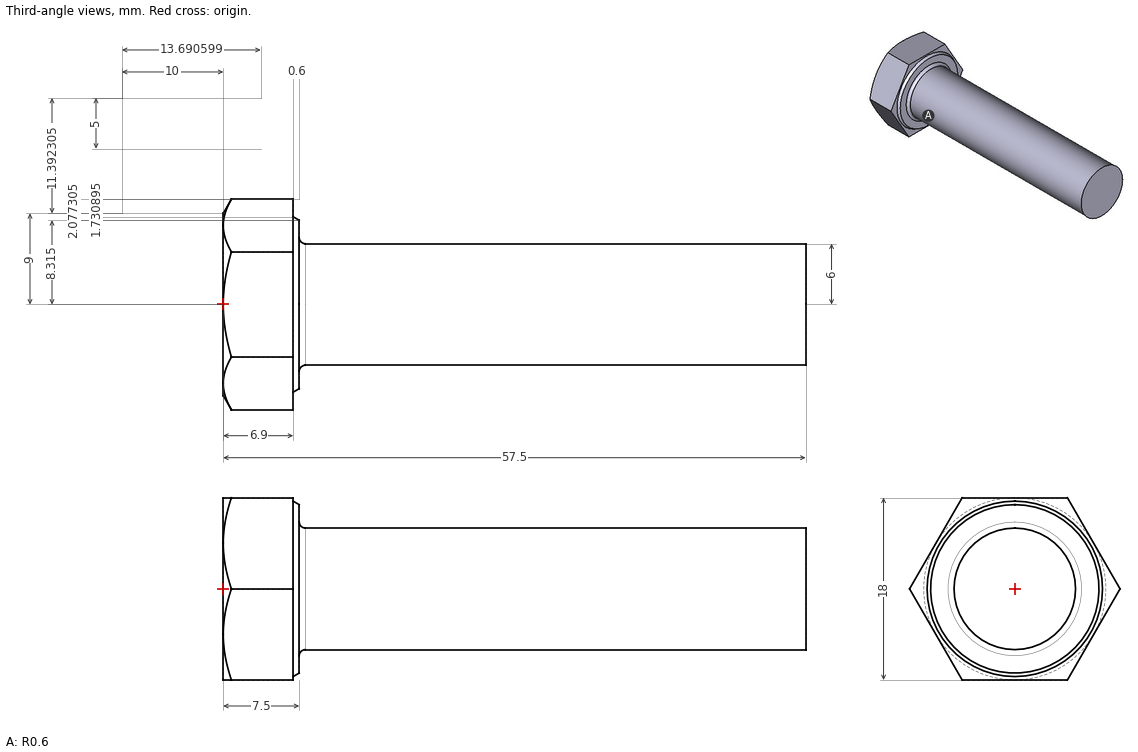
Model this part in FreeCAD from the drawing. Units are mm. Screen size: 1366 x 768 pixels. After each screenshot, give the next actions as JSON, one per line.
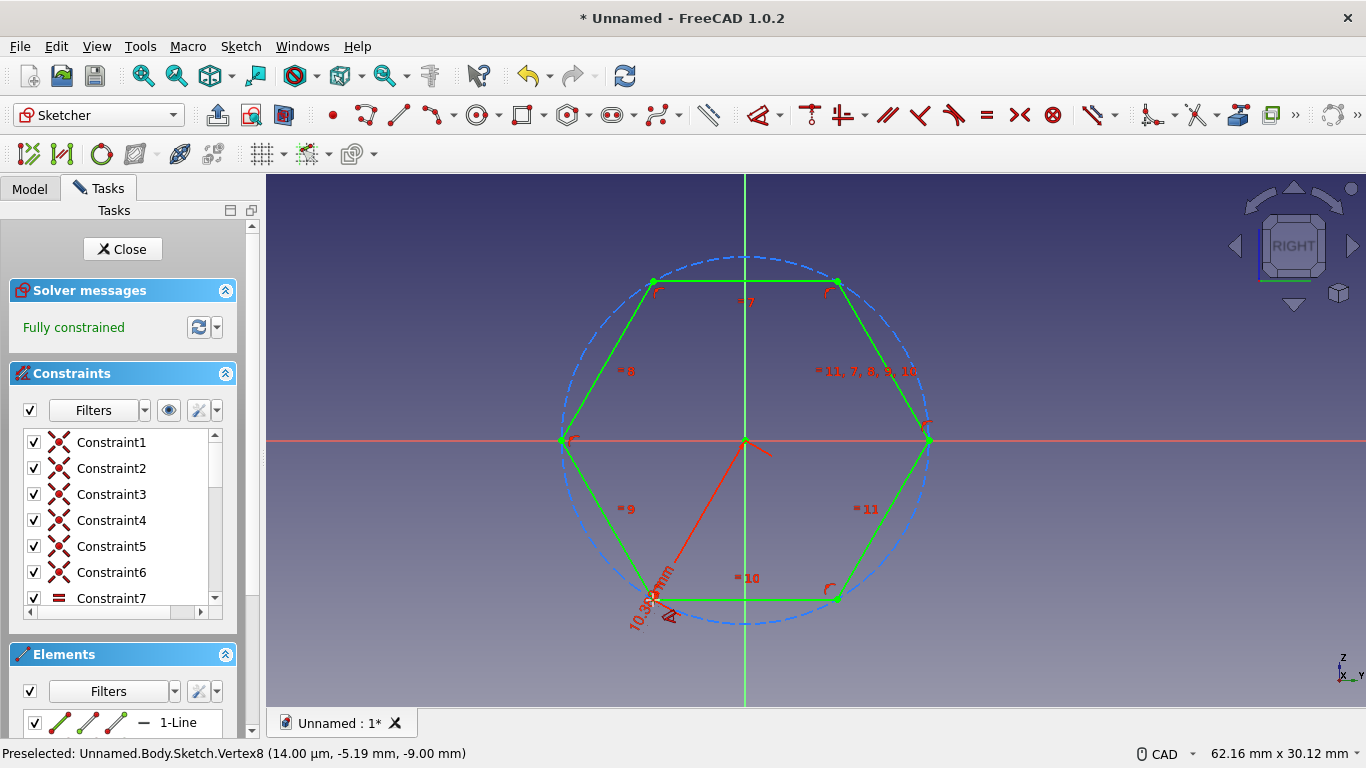
{"action": "left_click", "coordinate": [837, 281]}
{"action": "left_click", "coordinate": [871, 367]}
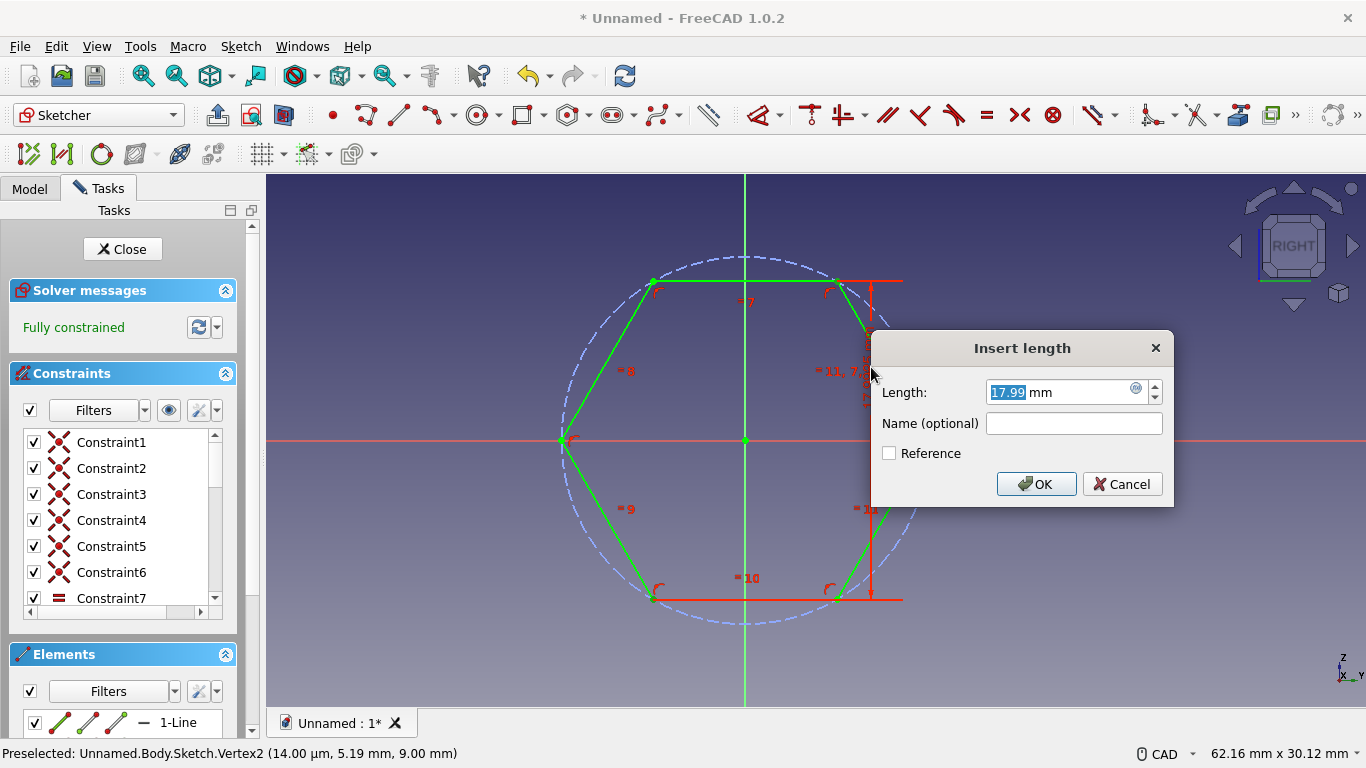
{"action": "type", "text": "18"}
{"action": "key", "text": "Return"}
{"action": "key", "text": "Escape"}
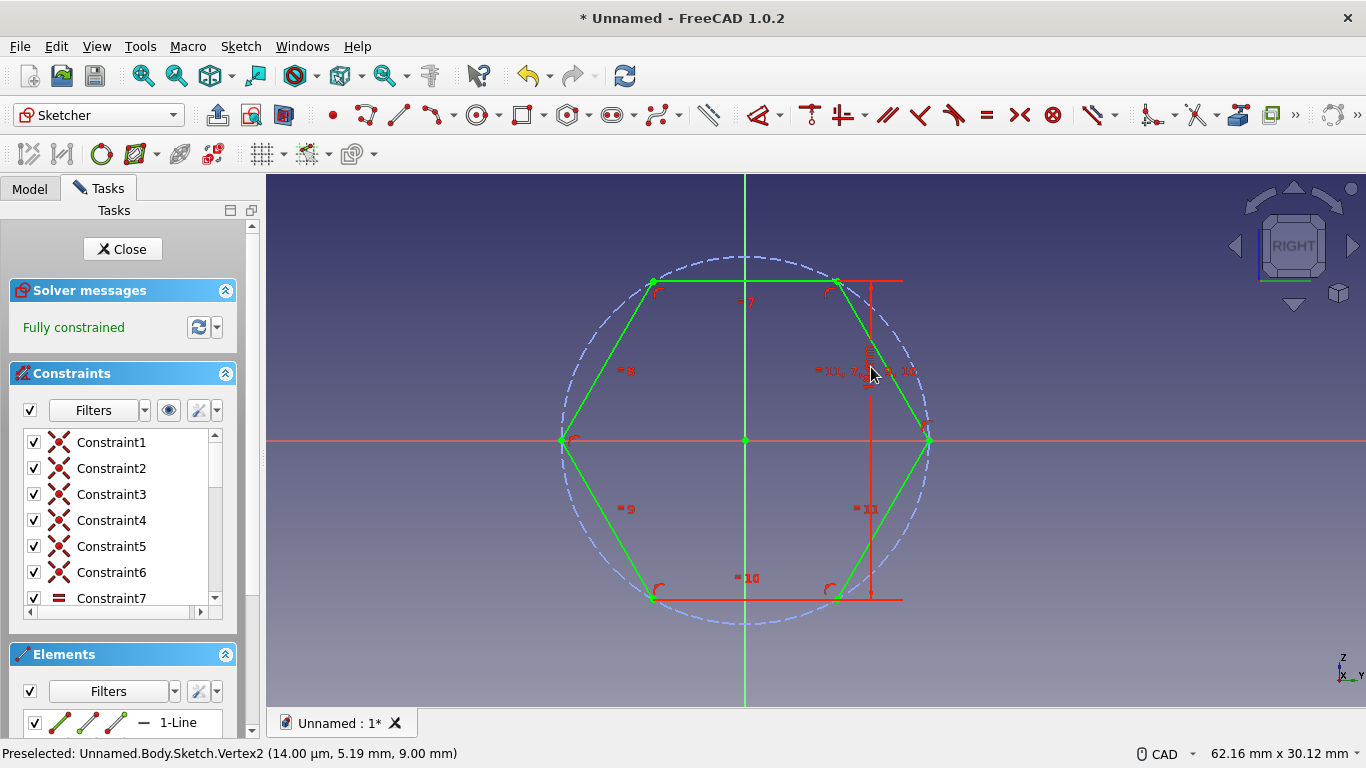
{"action": "left_click", "coordinate": [123, 249]}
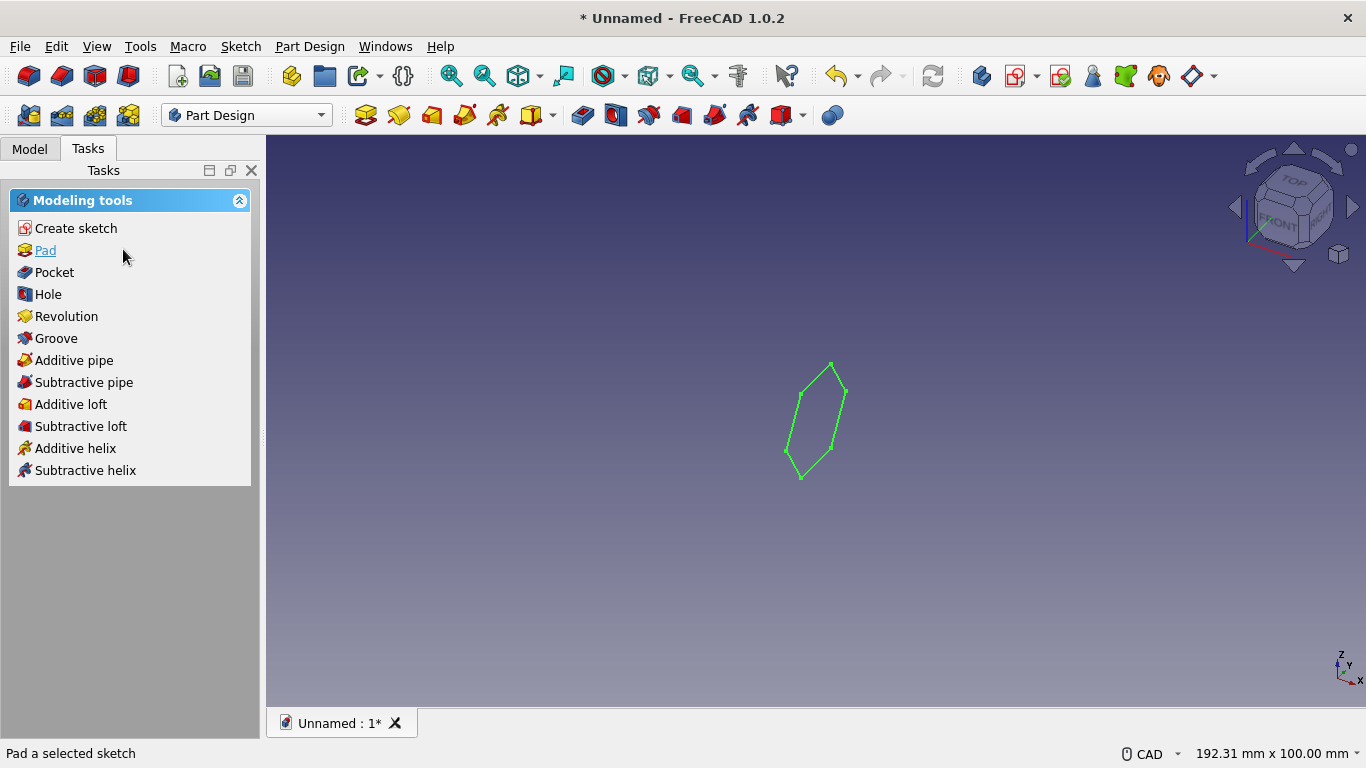
{"action": "left_click", "coordinate": [366, 116]}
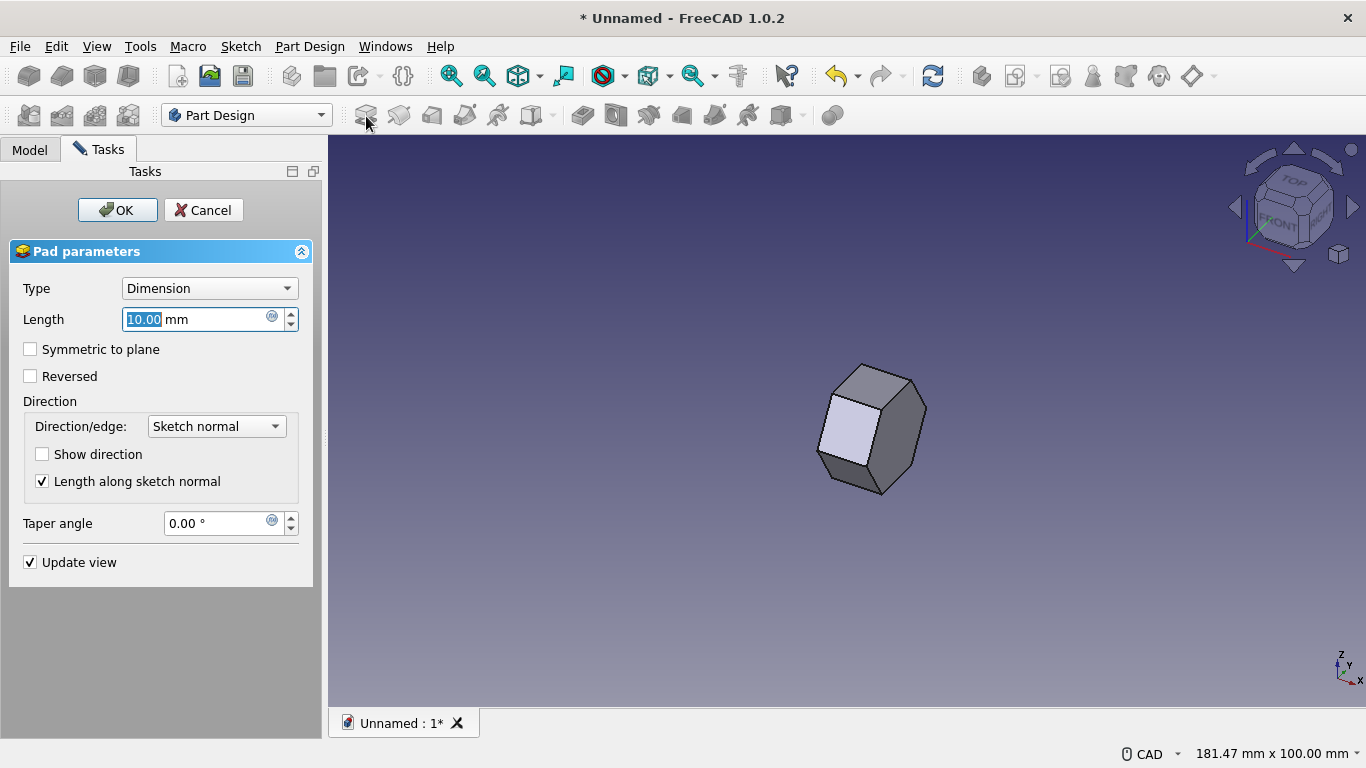
{"action": "type", "text": "7.5"}
{"action": "key", "text": "Tab"}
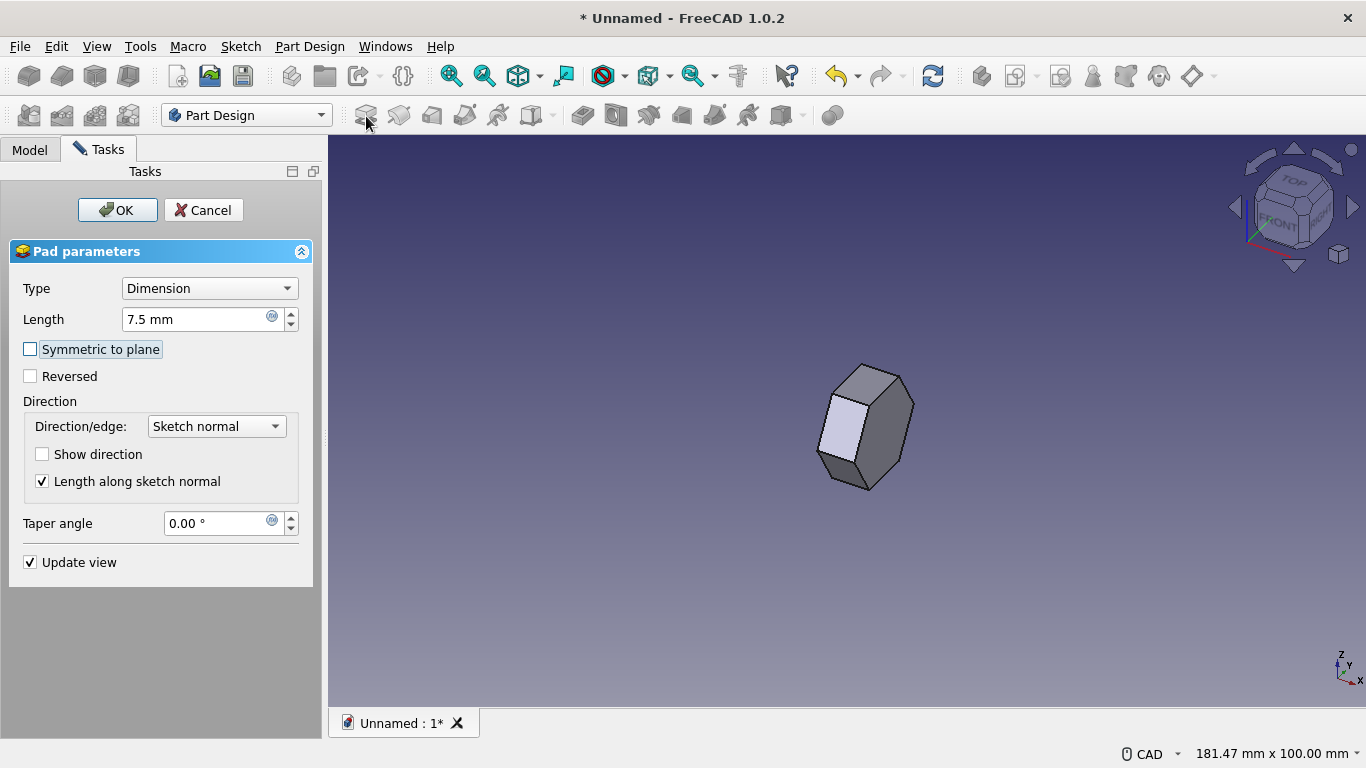
{"action": "left_click", "coordinate": [118, 210]}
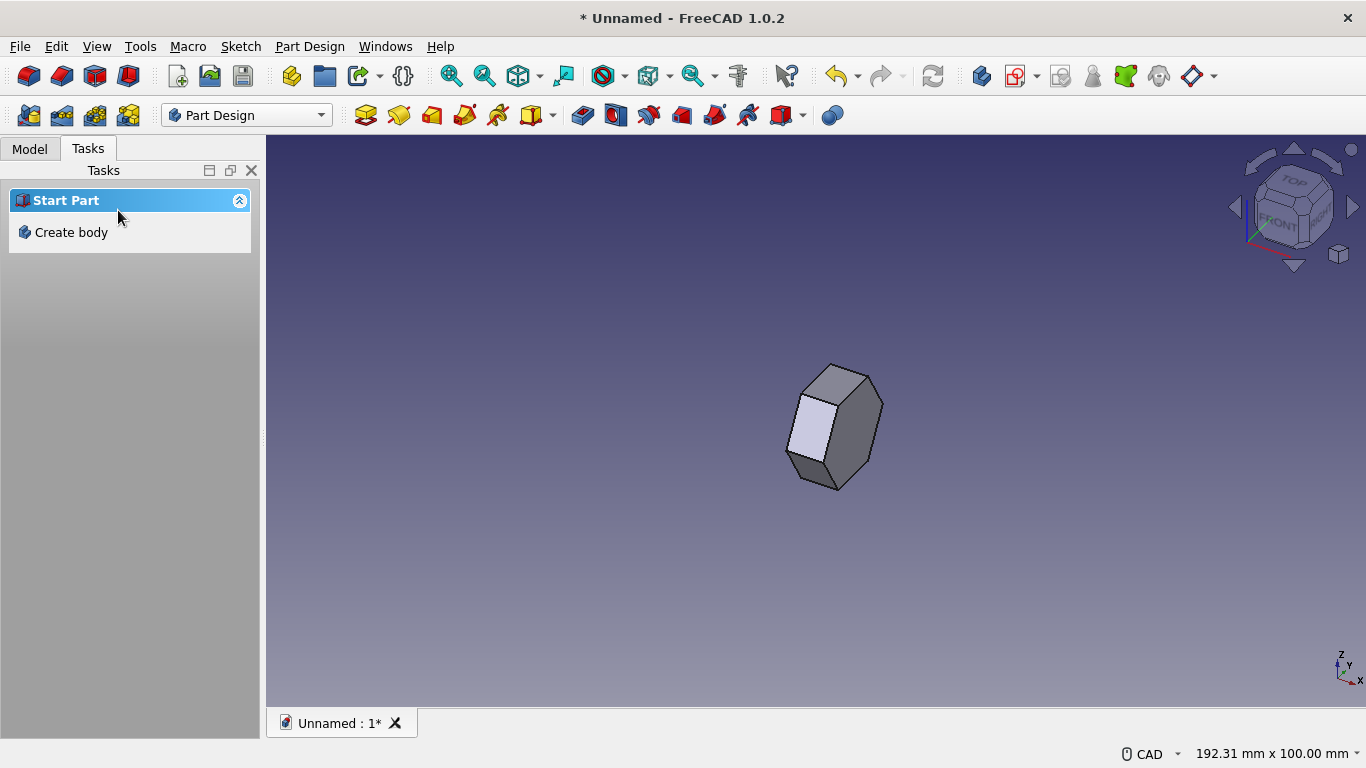
{"action": "left_click", "coordinate": [452, 76]}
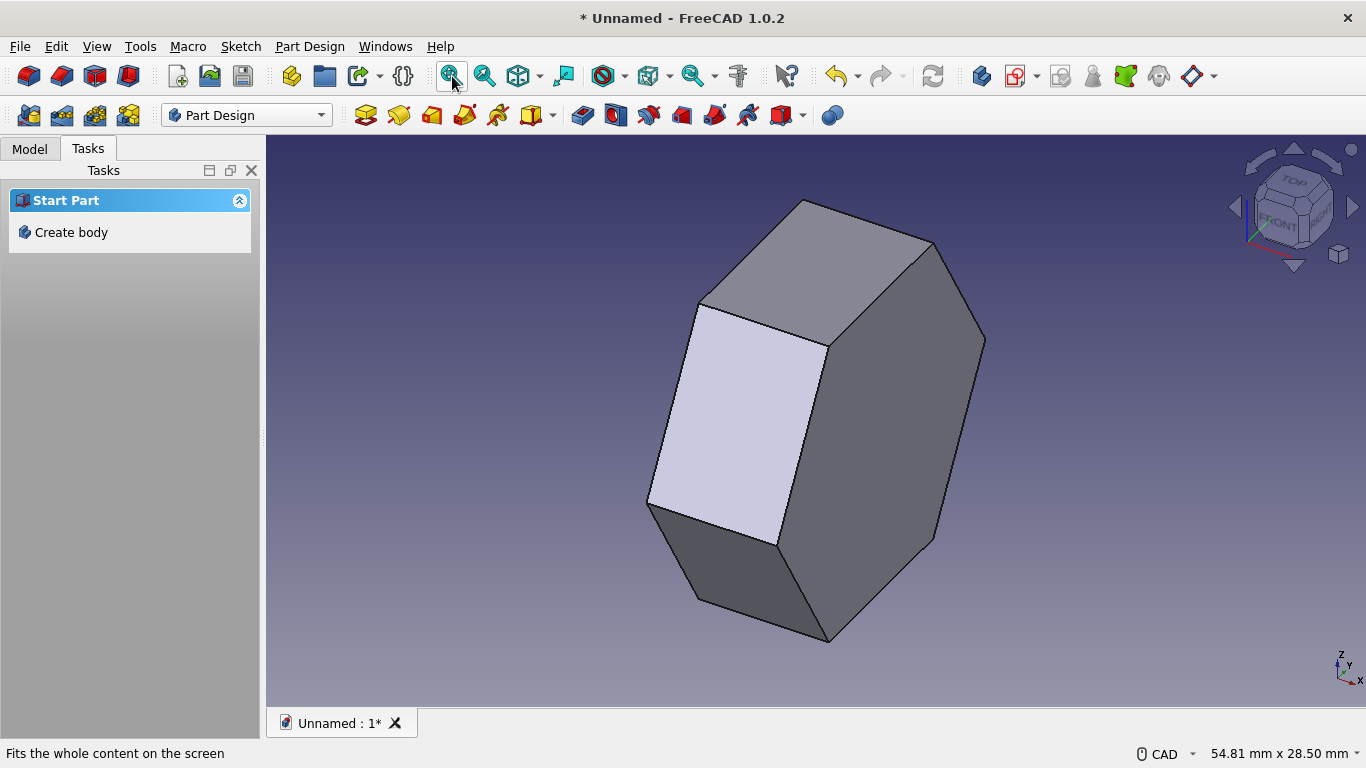
{"action": "left_click", "coordinate": [1014, 76]}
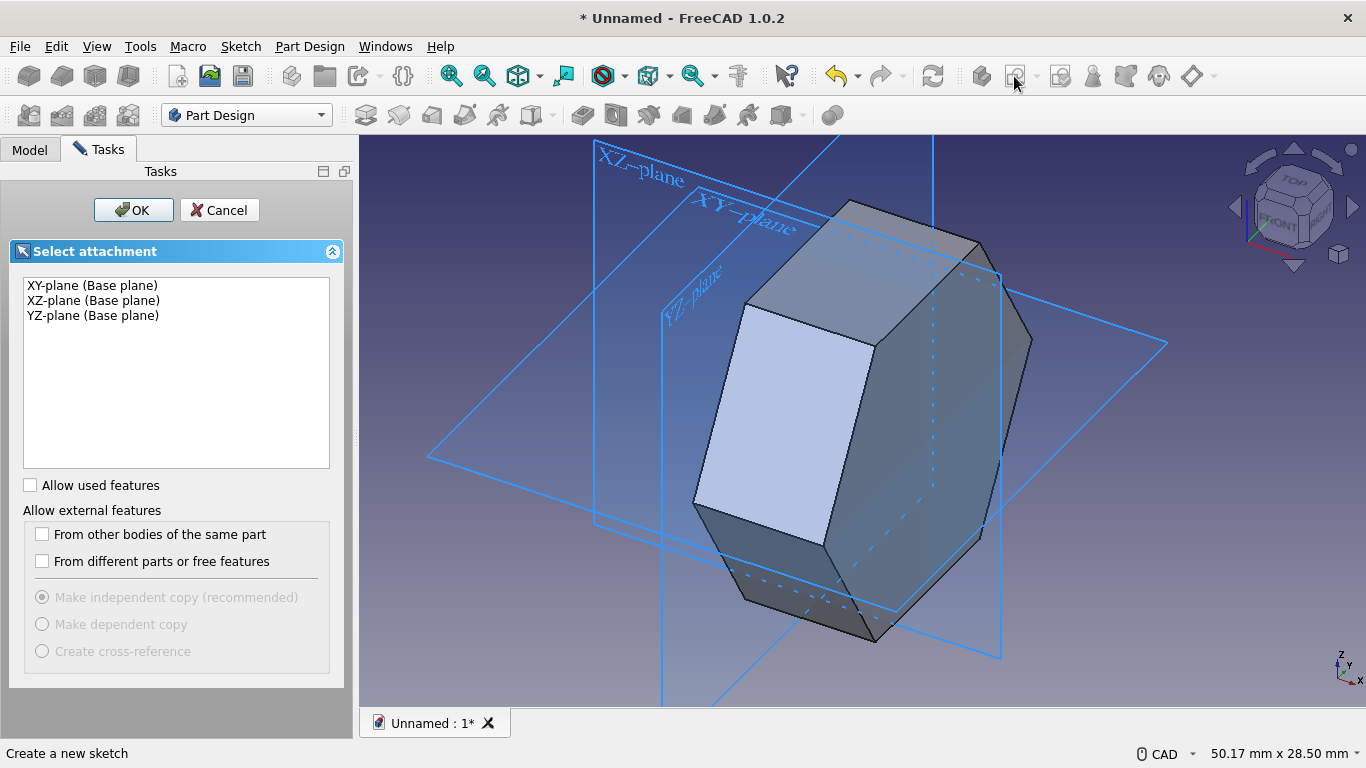
{"action": "left_click", "coordinate": [84, 286]}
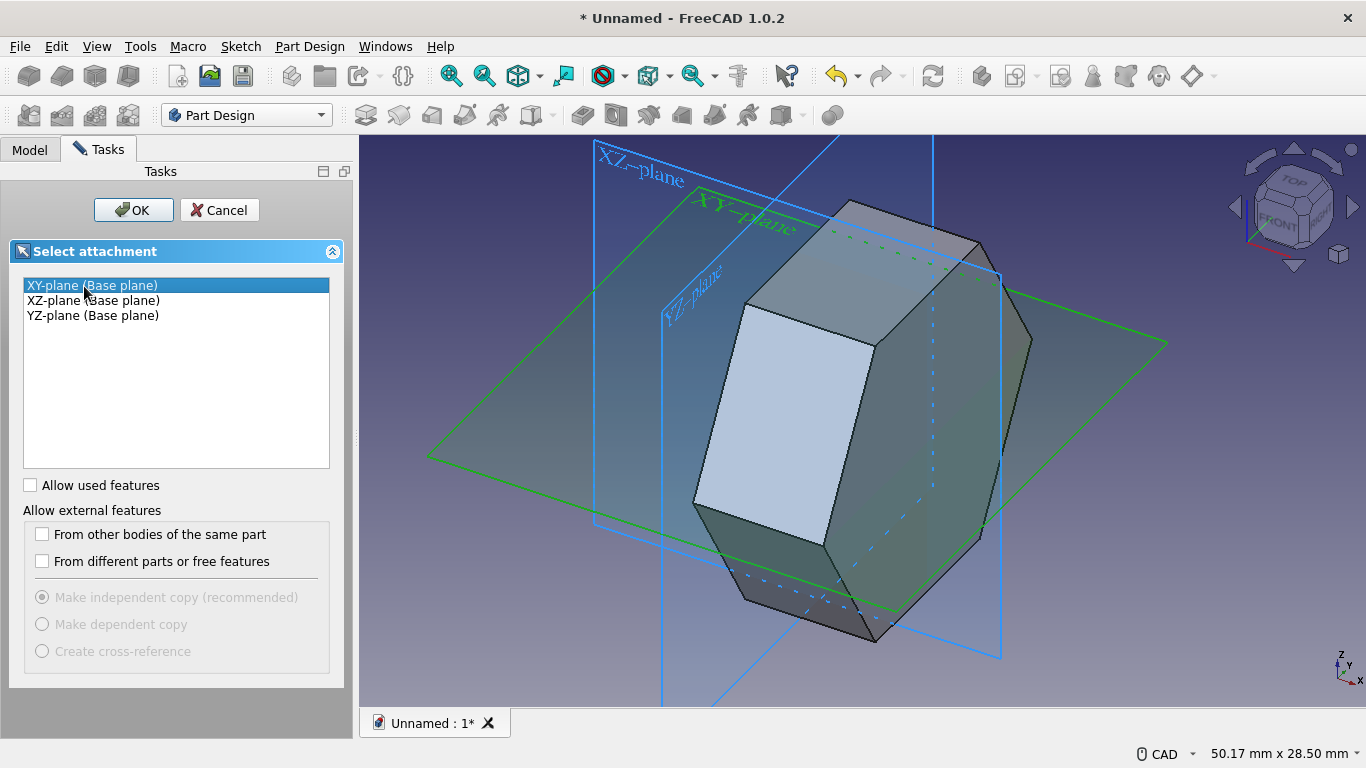
{"action": "left_click", "coordinate": [134, 210]}